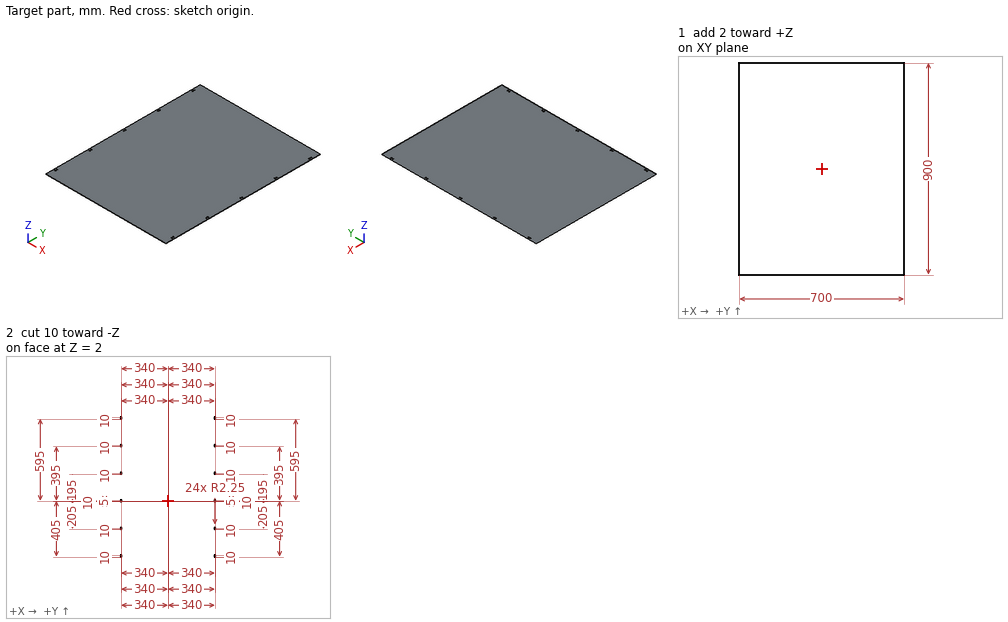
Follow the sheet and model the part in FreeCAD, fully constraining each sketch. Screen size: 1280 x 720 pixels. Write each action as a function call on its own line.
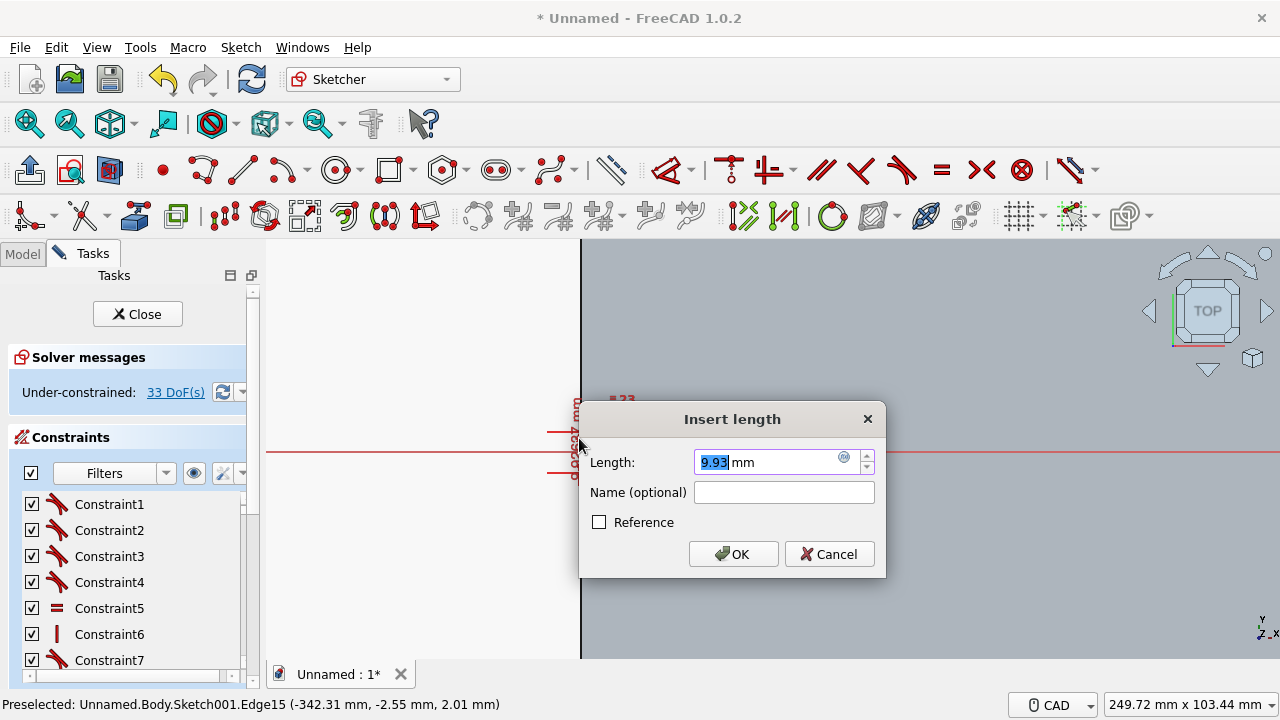
text(10)
key(Return)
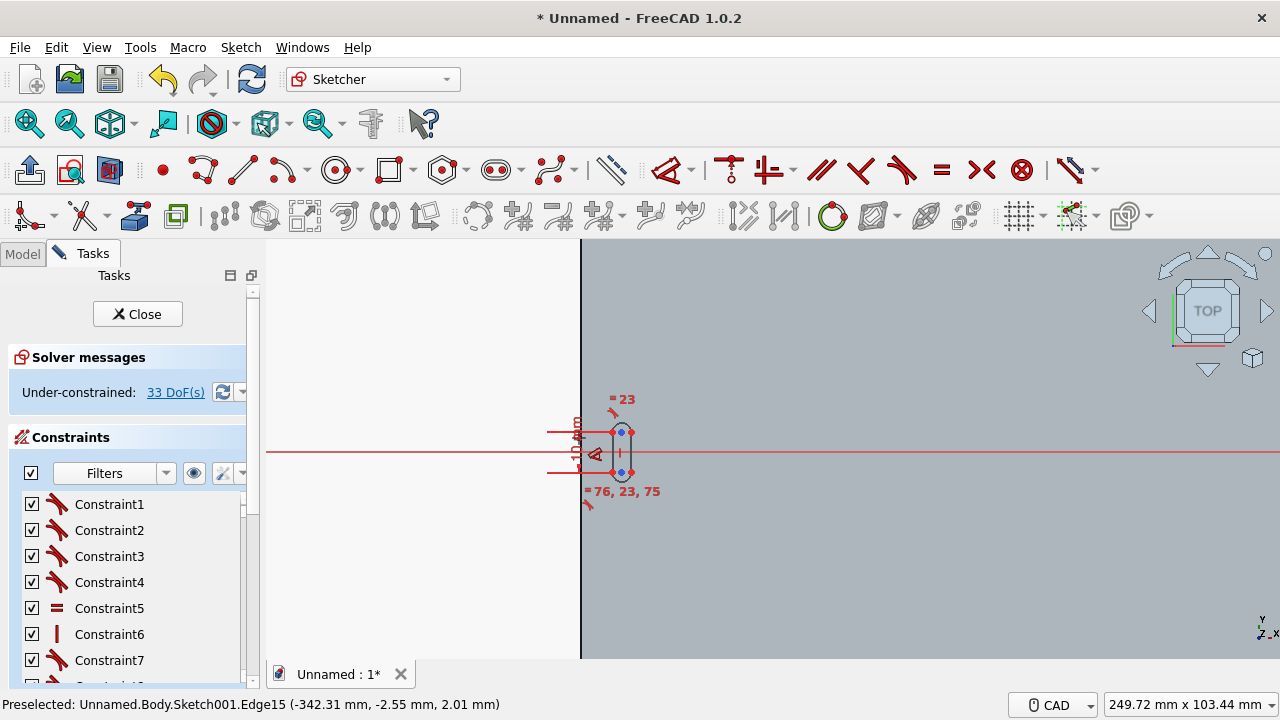
scroll(620, 475, down, 14)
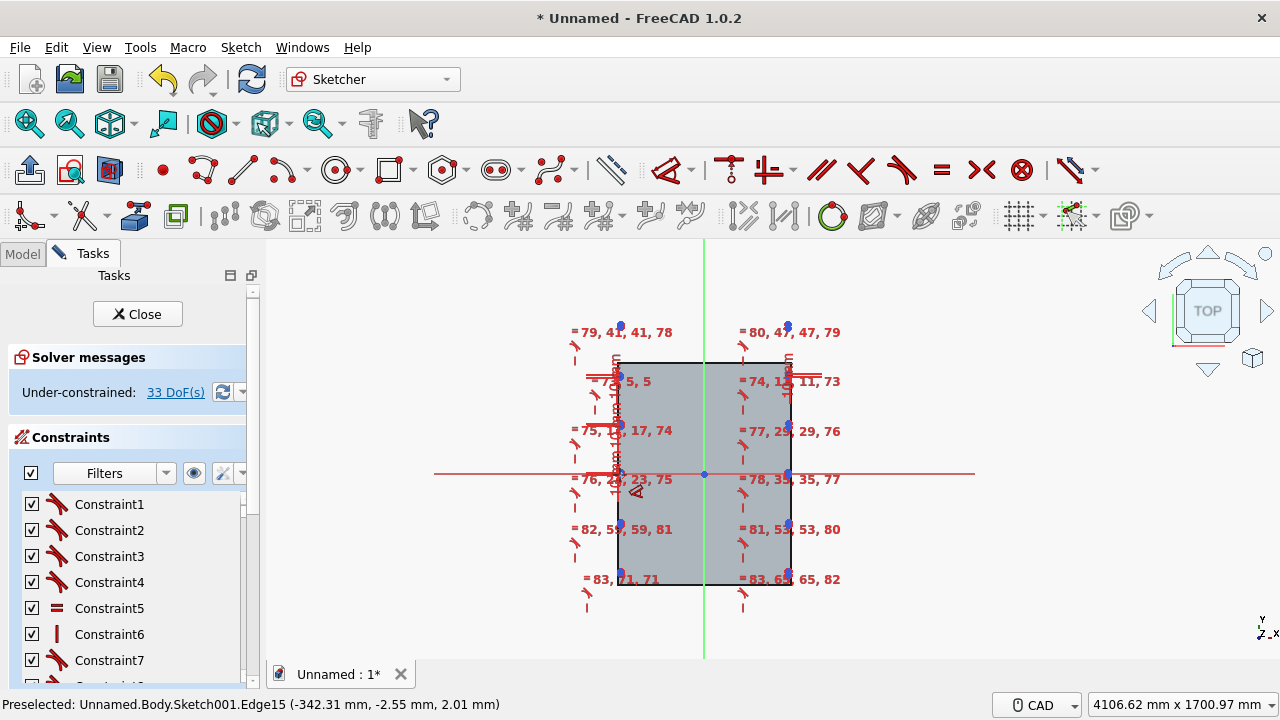
scroll(788, 426, up, 14)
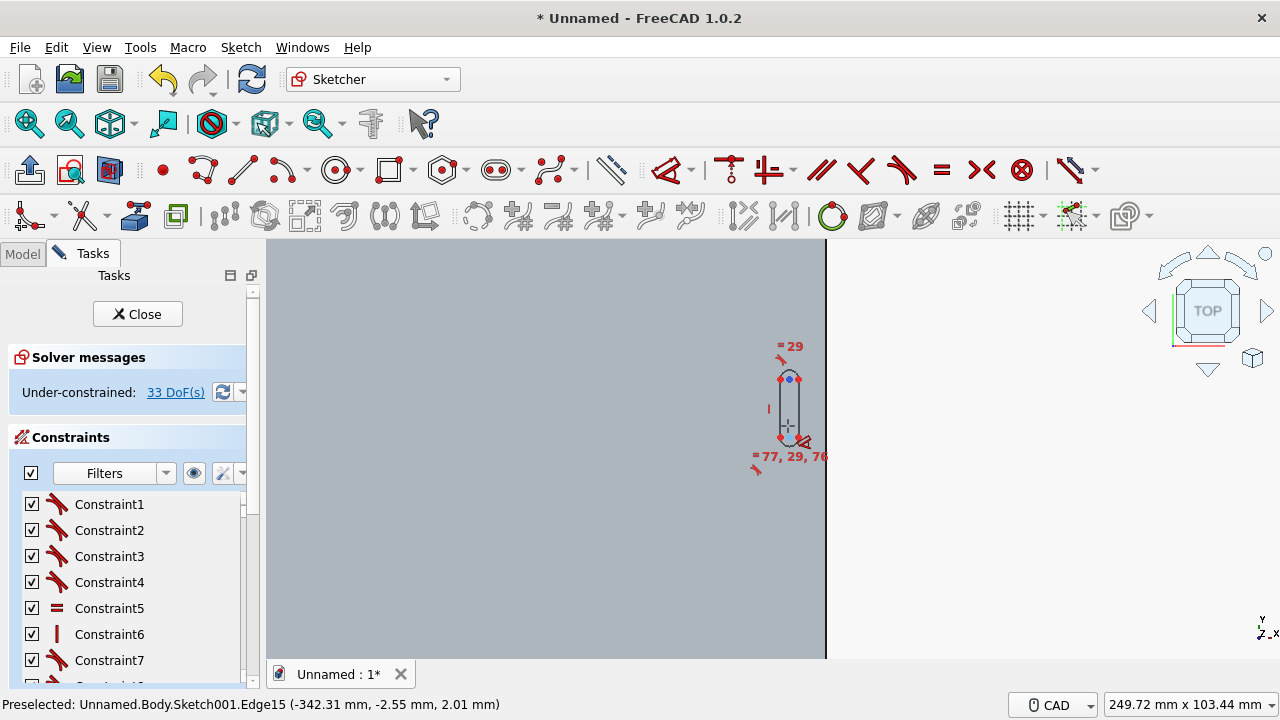
click(780, 420)
click(814, 408)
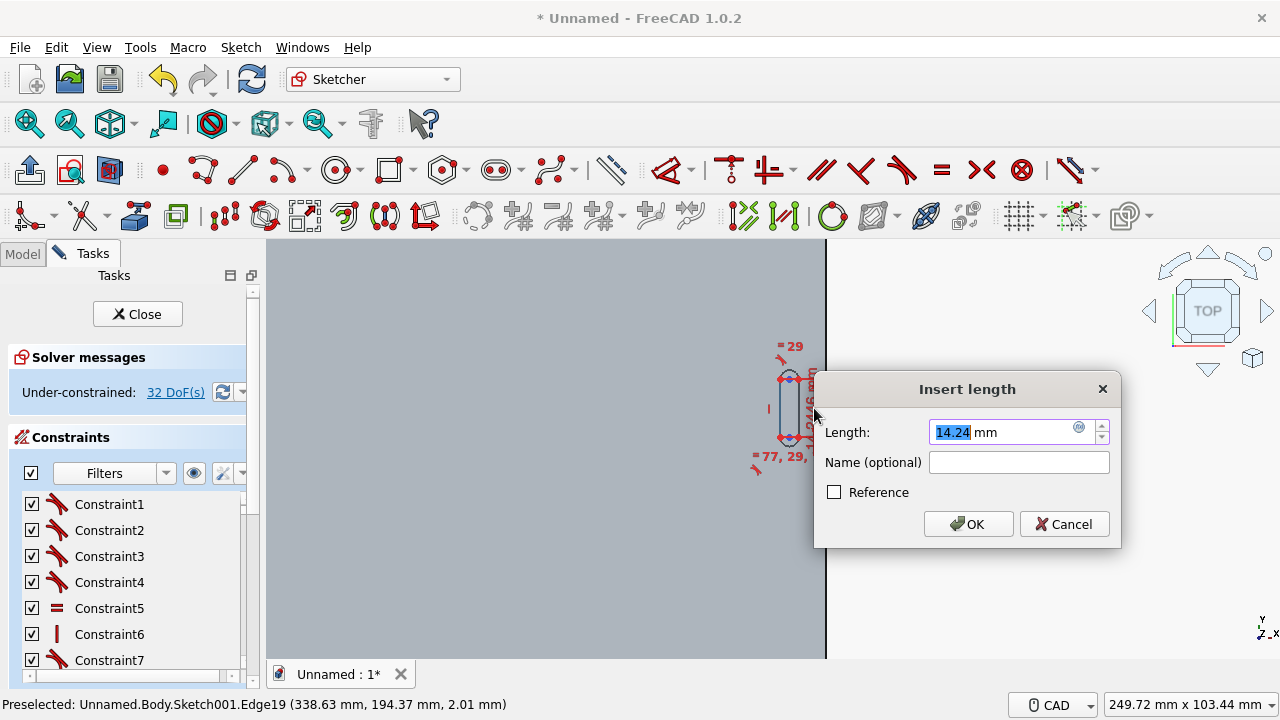
text(10)
key(Return)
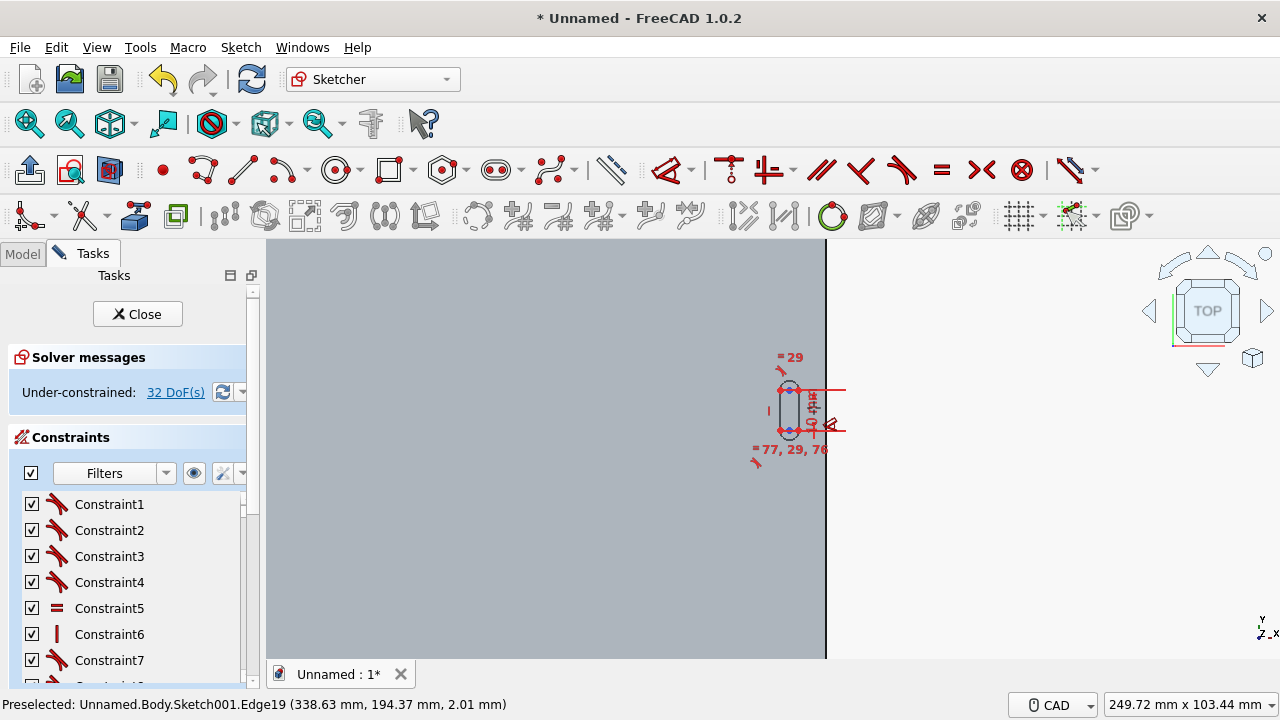
scroll(789, 426, down, 14)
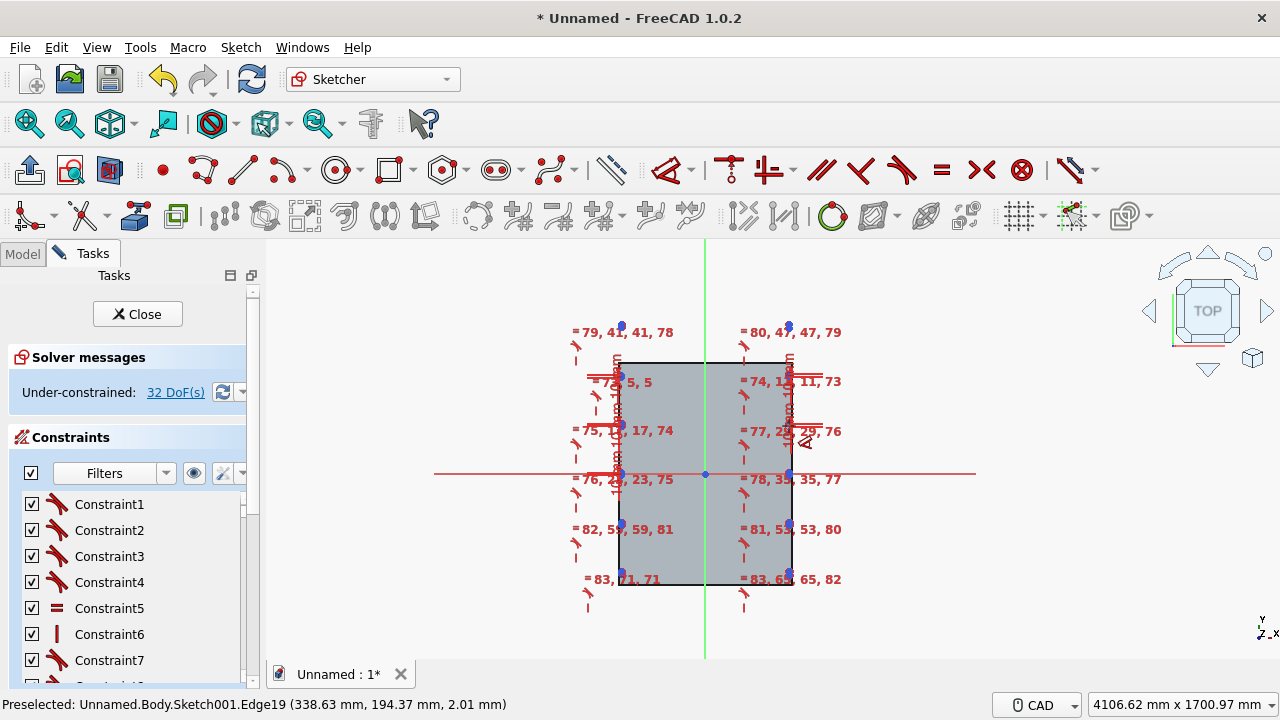
scroll(789, 475, up, 14)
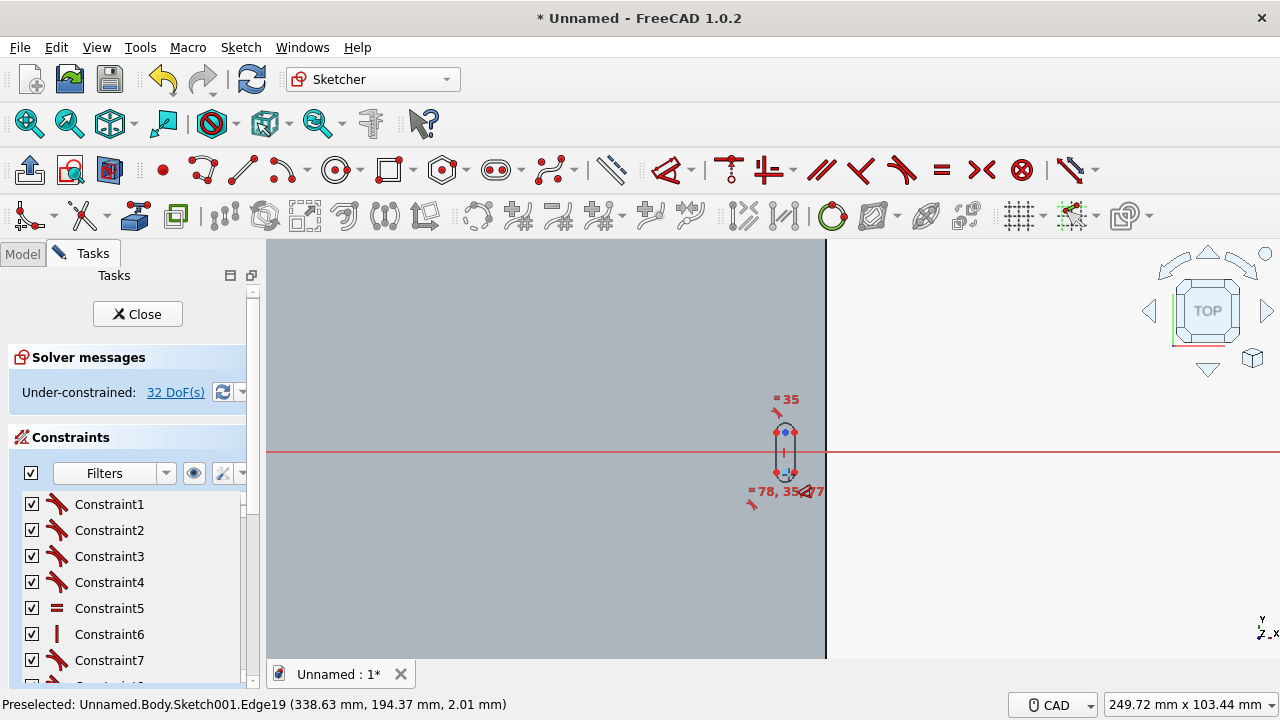
click(776, 461)
click(810, 438)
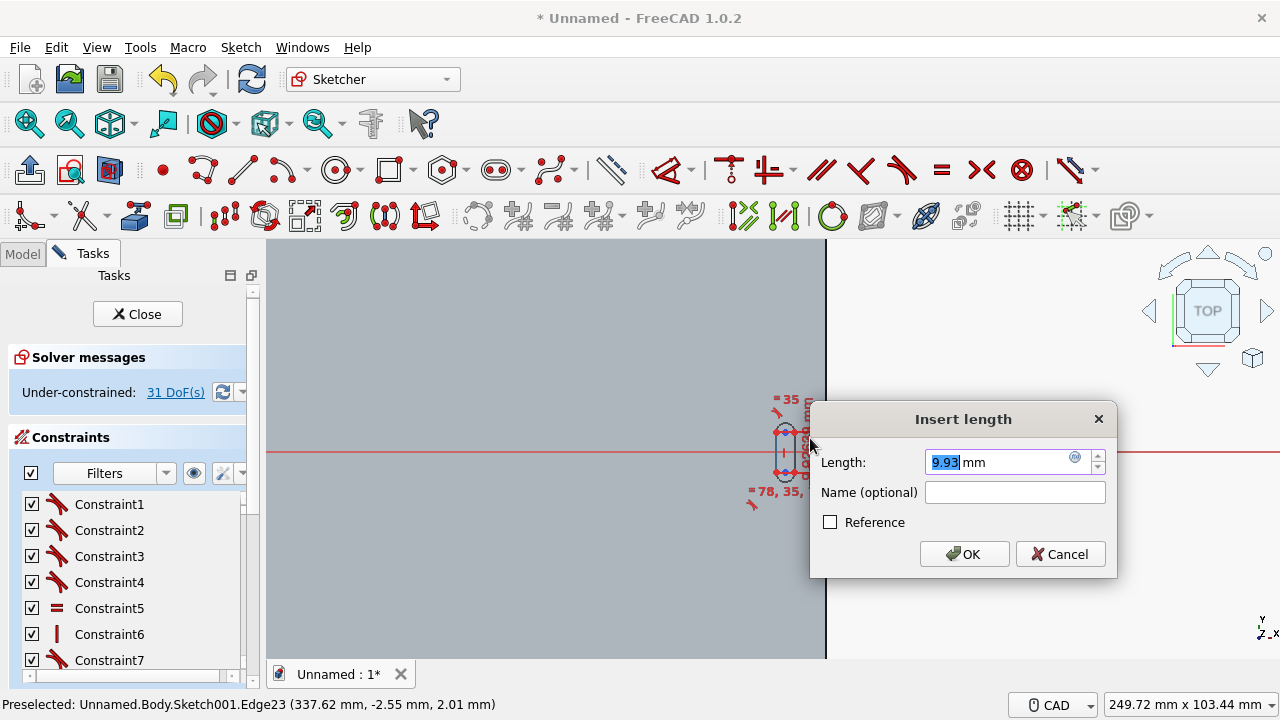
text(10)
key(Return)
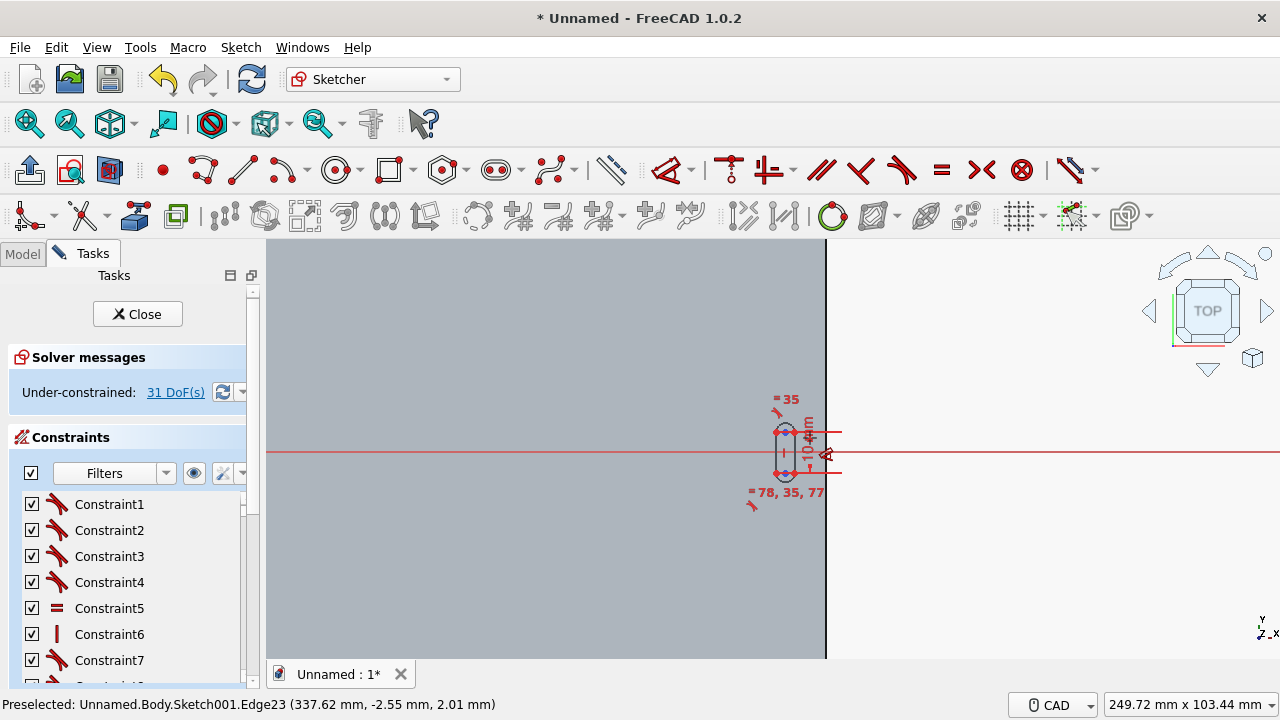
scroll(789, 475, down, 14)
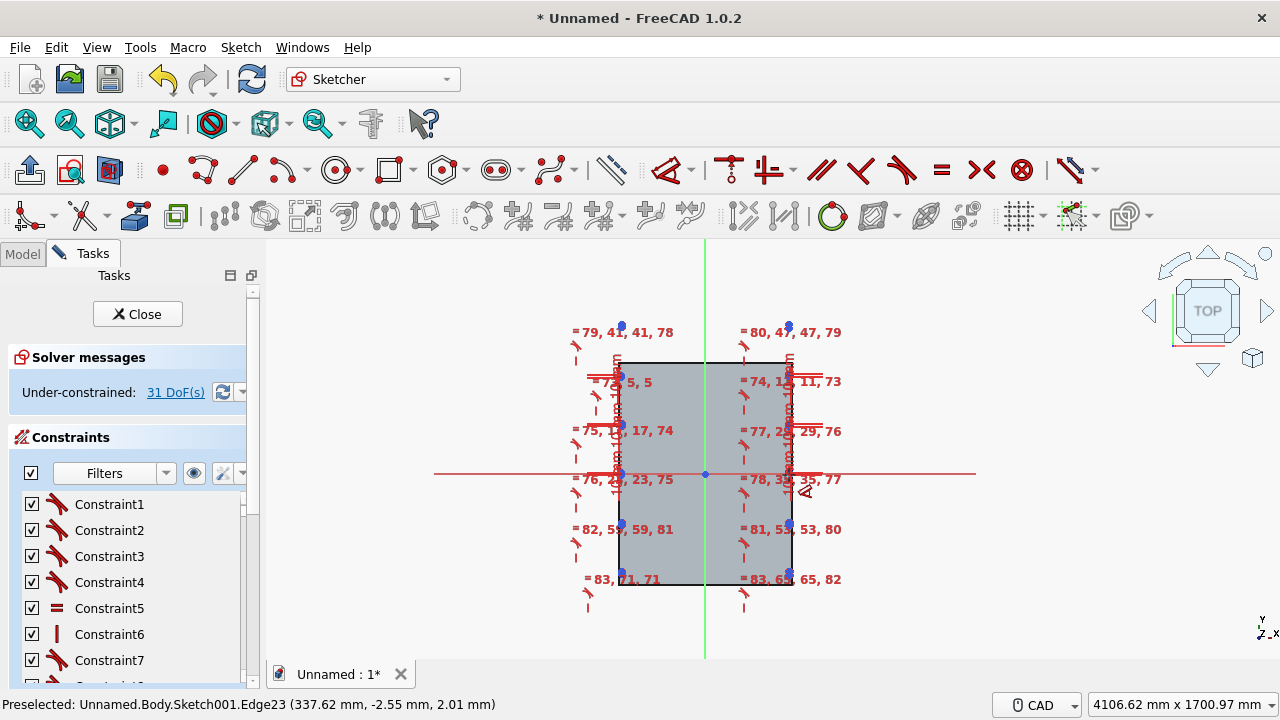
scroll(621, 327, up, 14)